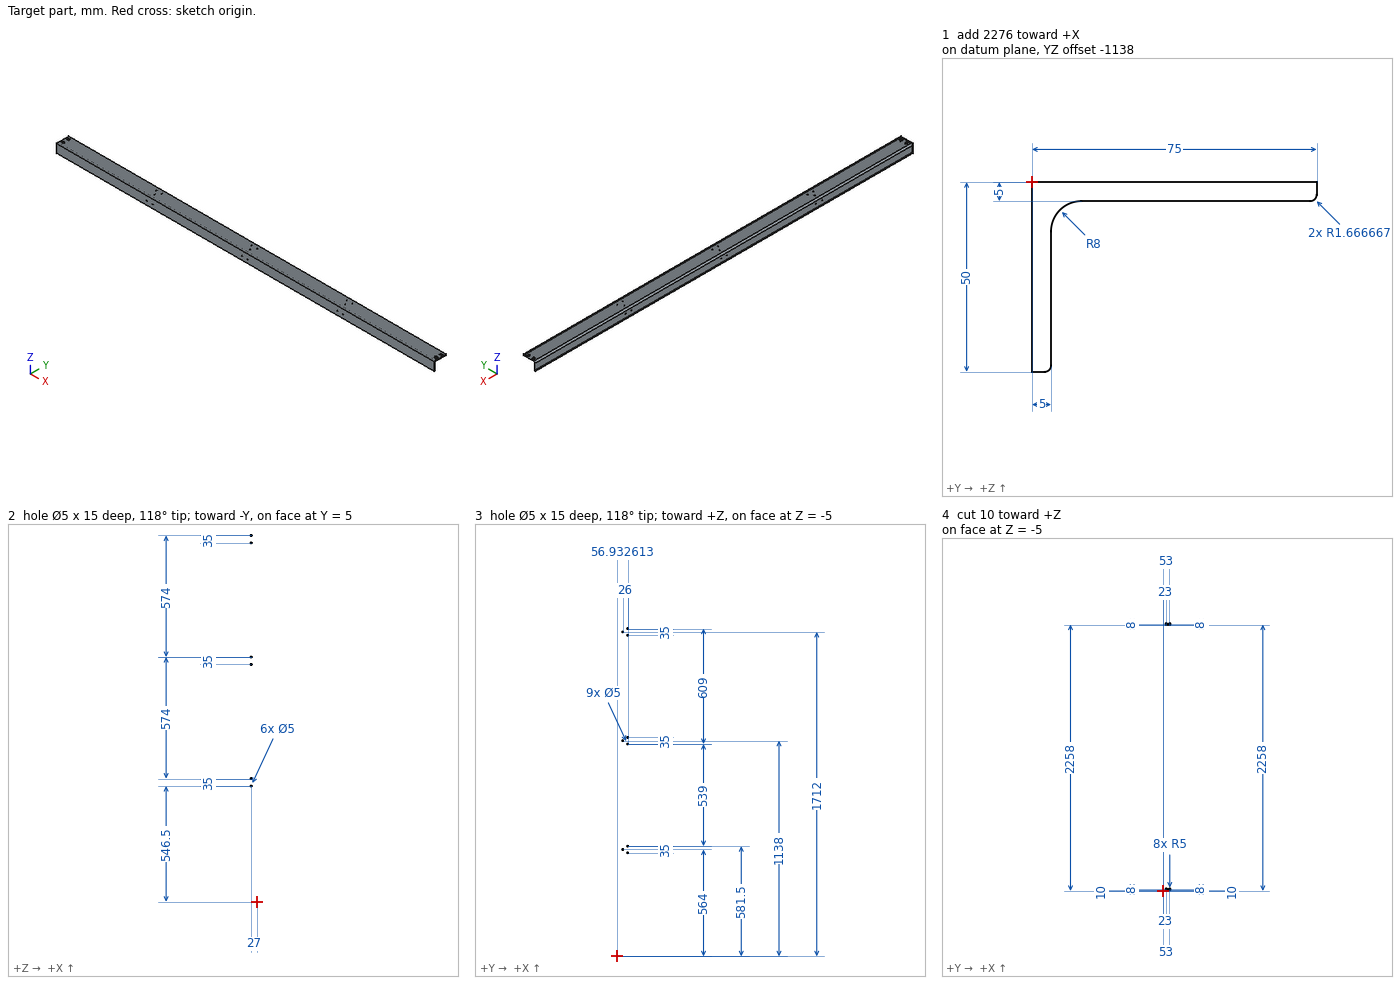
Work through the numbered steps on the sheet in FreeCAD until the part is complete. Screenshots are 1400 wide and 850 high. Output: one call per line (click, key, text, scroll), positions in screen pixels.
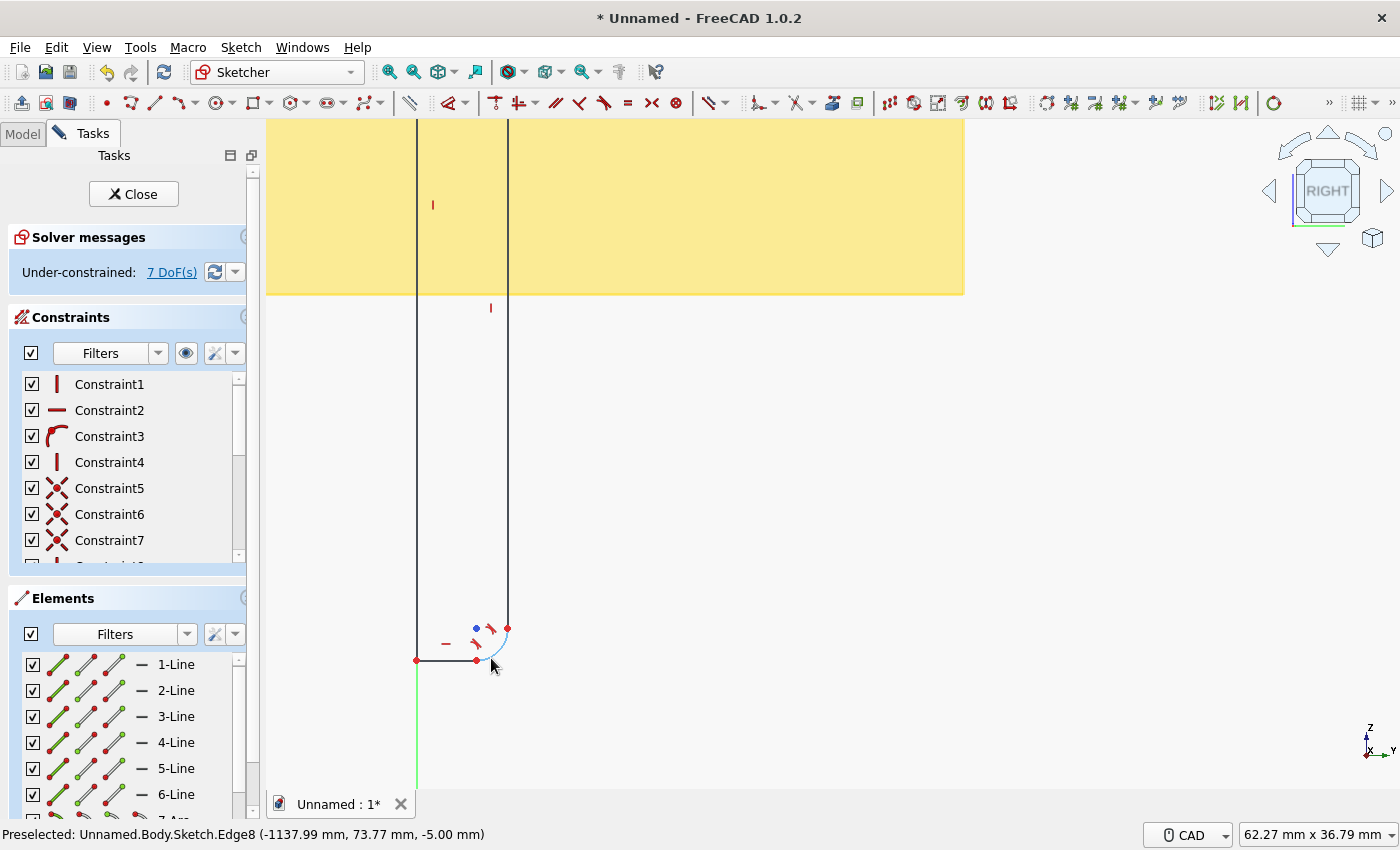
click(490, 657)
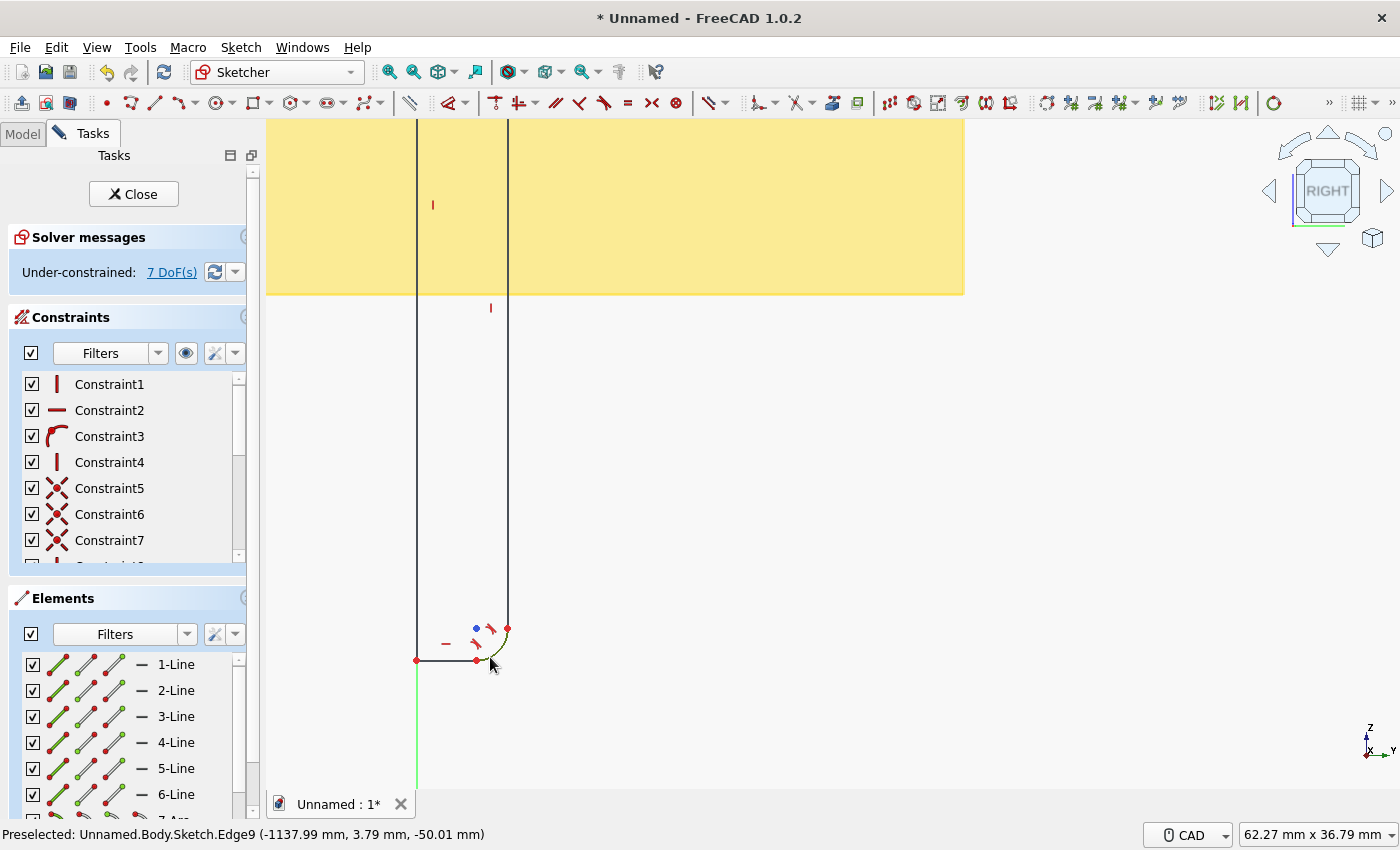
click(628, 104)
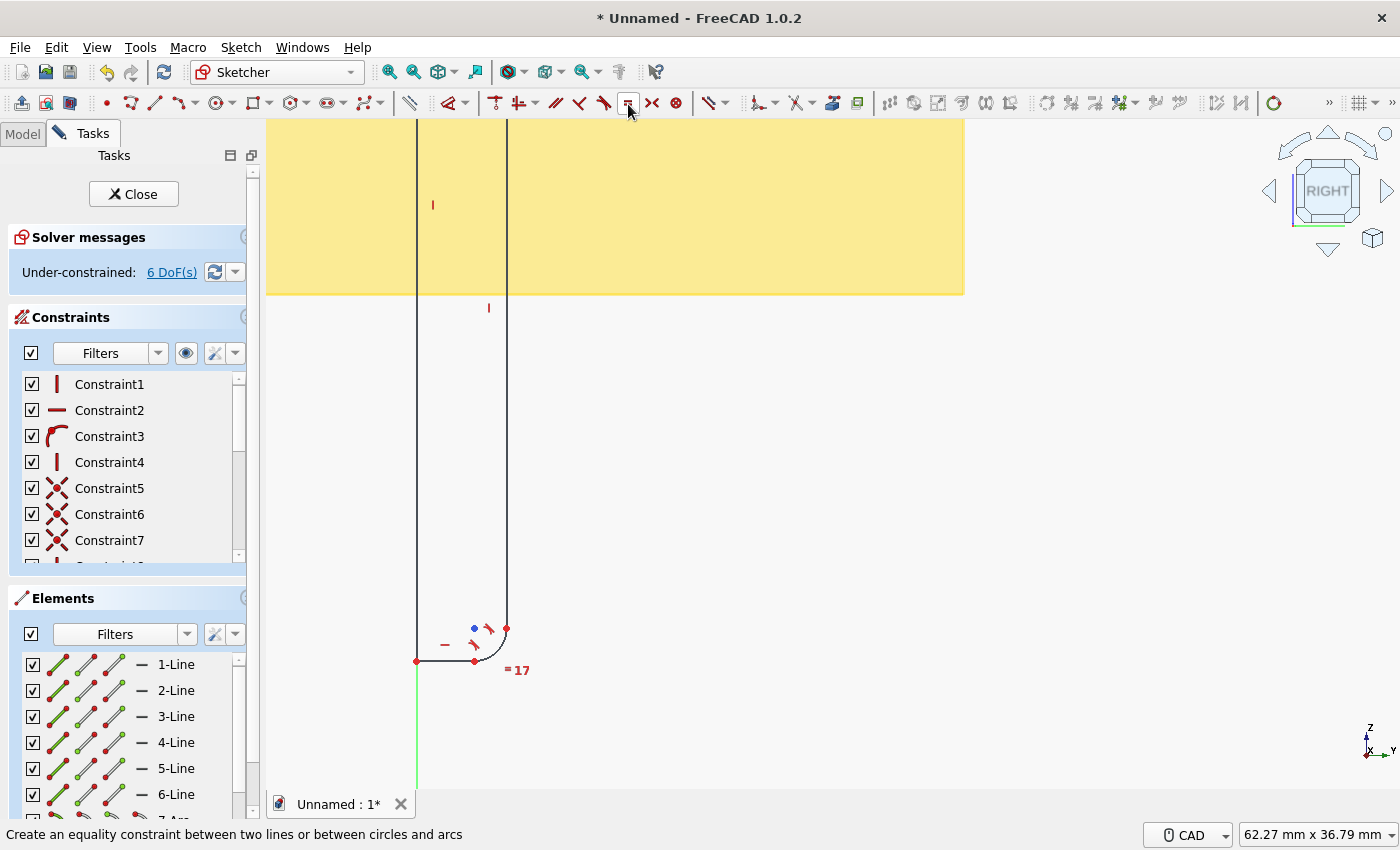
click(448, 104)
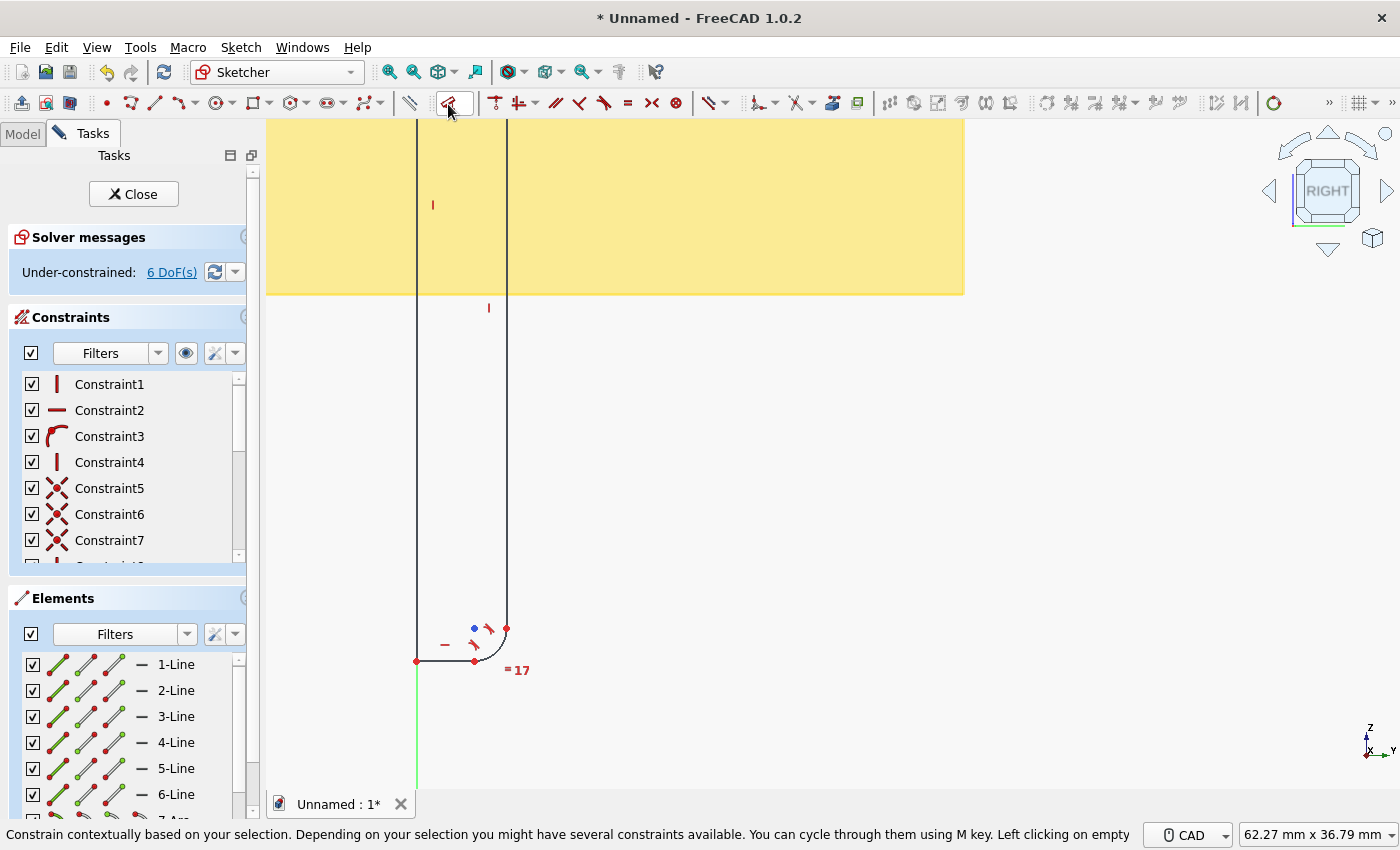
scroll(491, 658, down, 4)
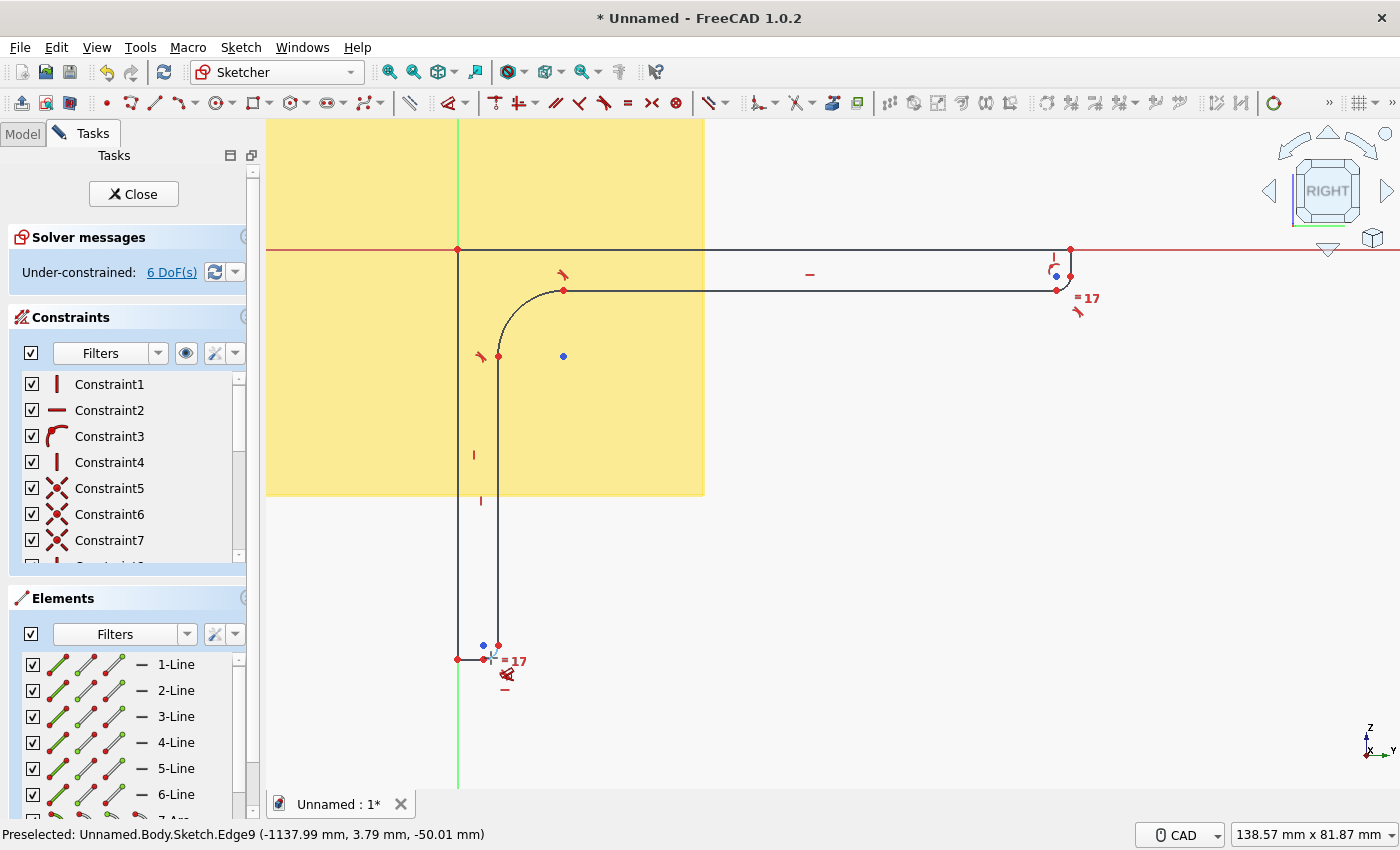
click(534, 298)
click(519, 270)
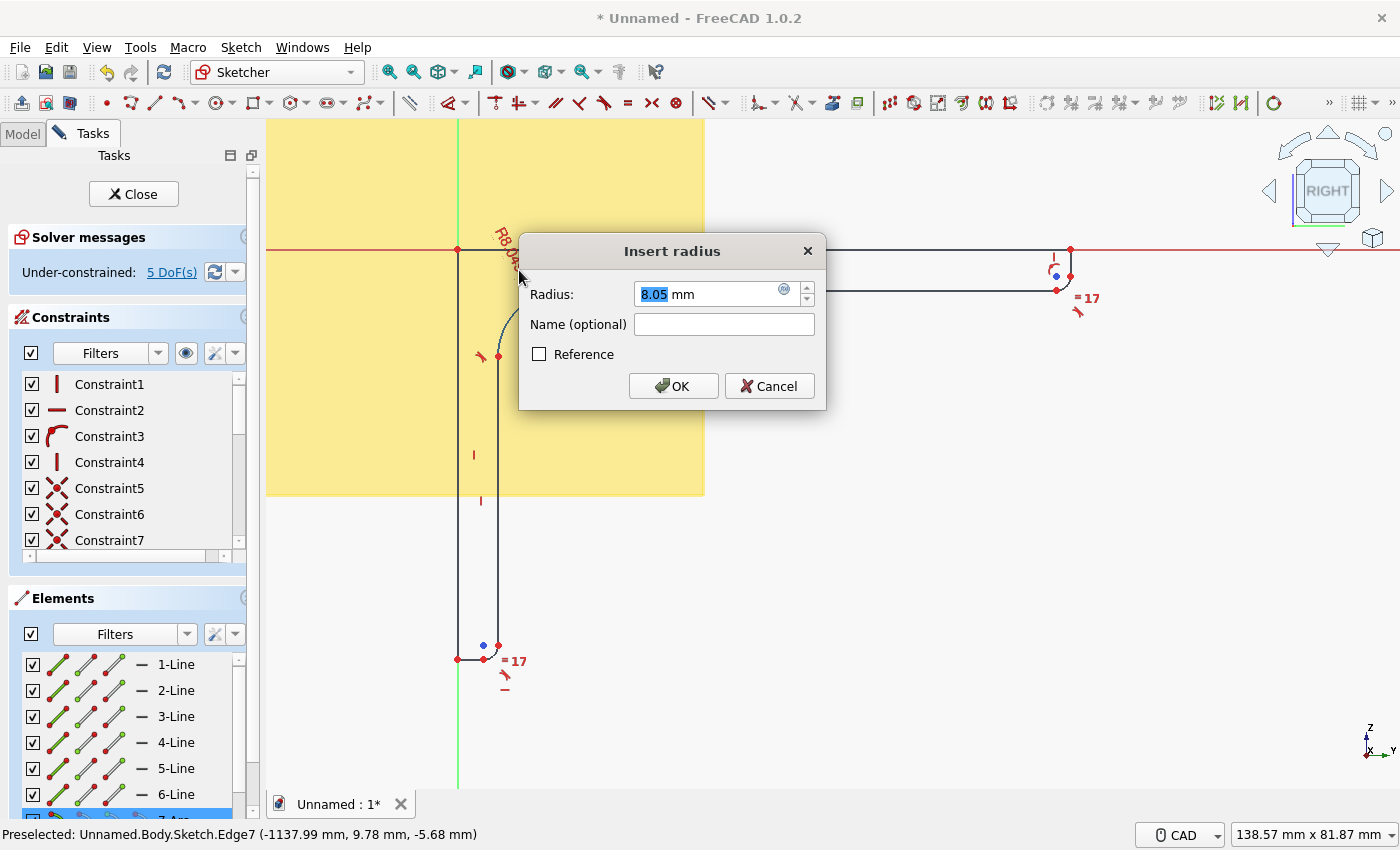
text(8)
key(Return)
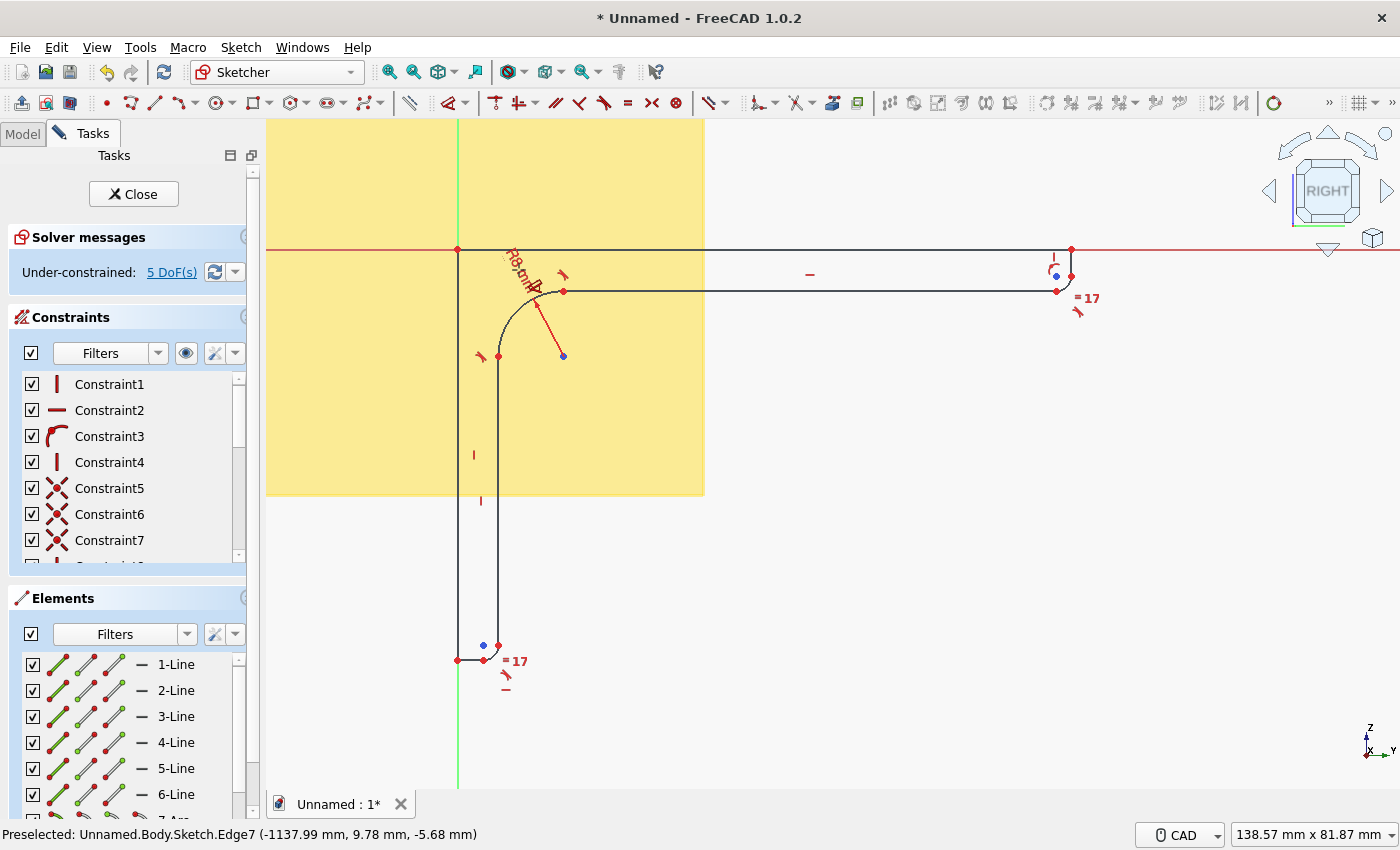
scroll(1067, 287, up, 6)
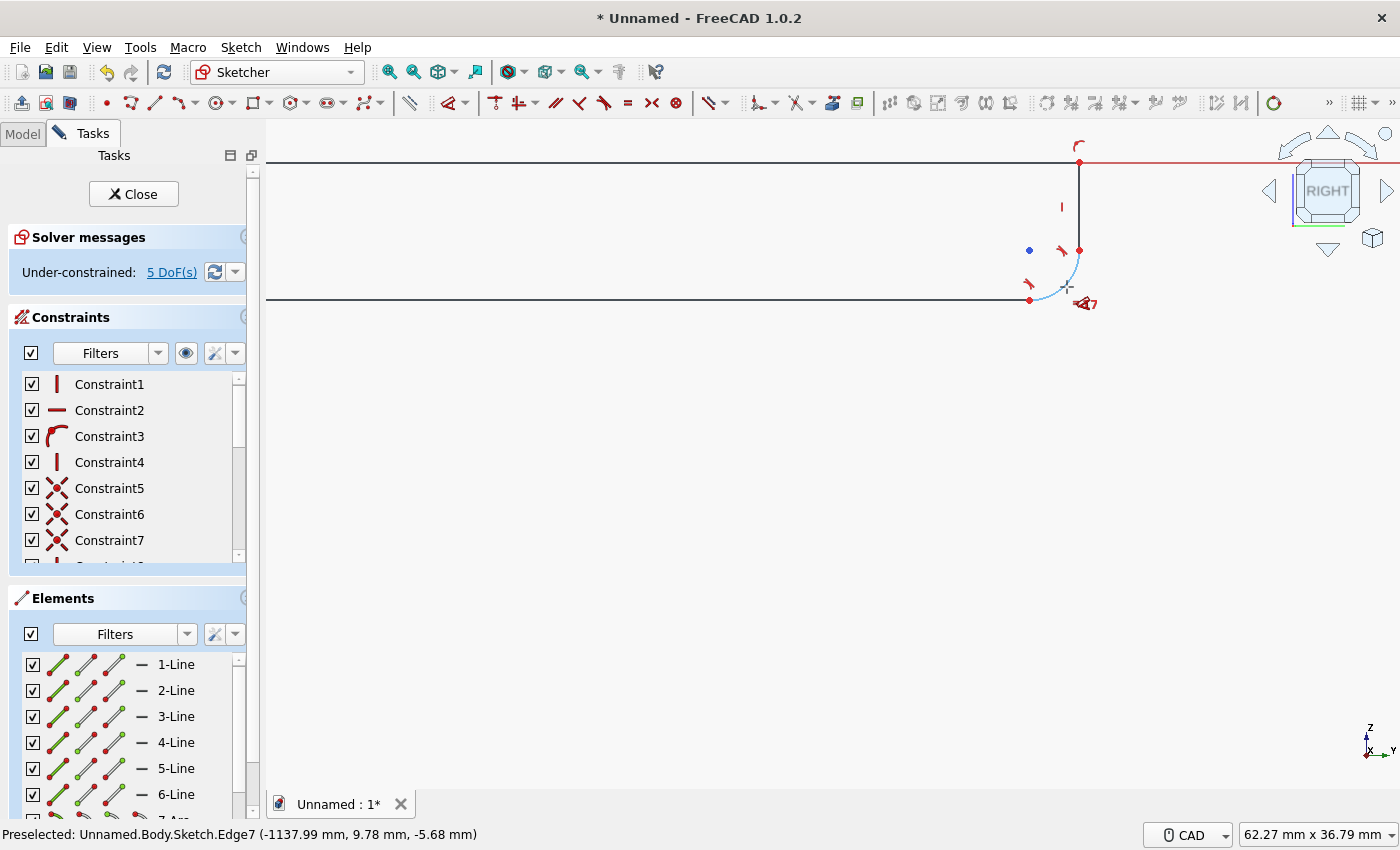
click(1065, 286)
click(1088, 309)